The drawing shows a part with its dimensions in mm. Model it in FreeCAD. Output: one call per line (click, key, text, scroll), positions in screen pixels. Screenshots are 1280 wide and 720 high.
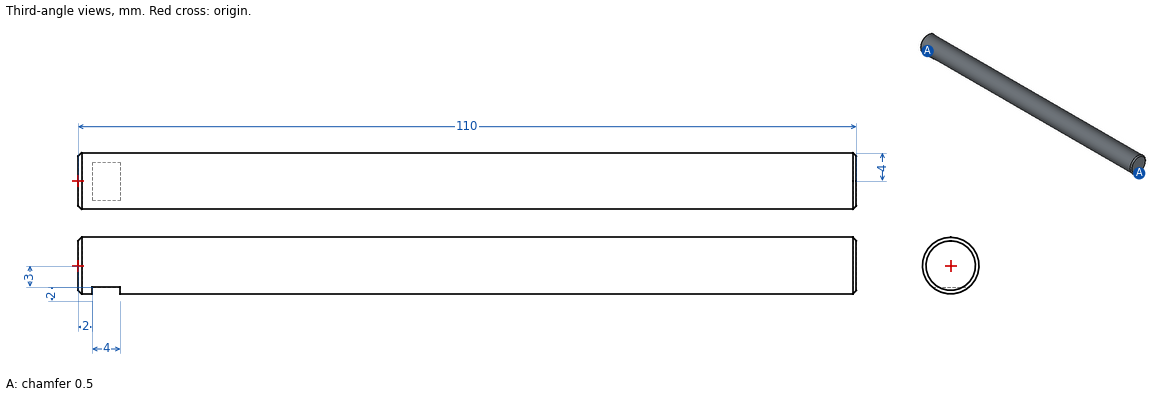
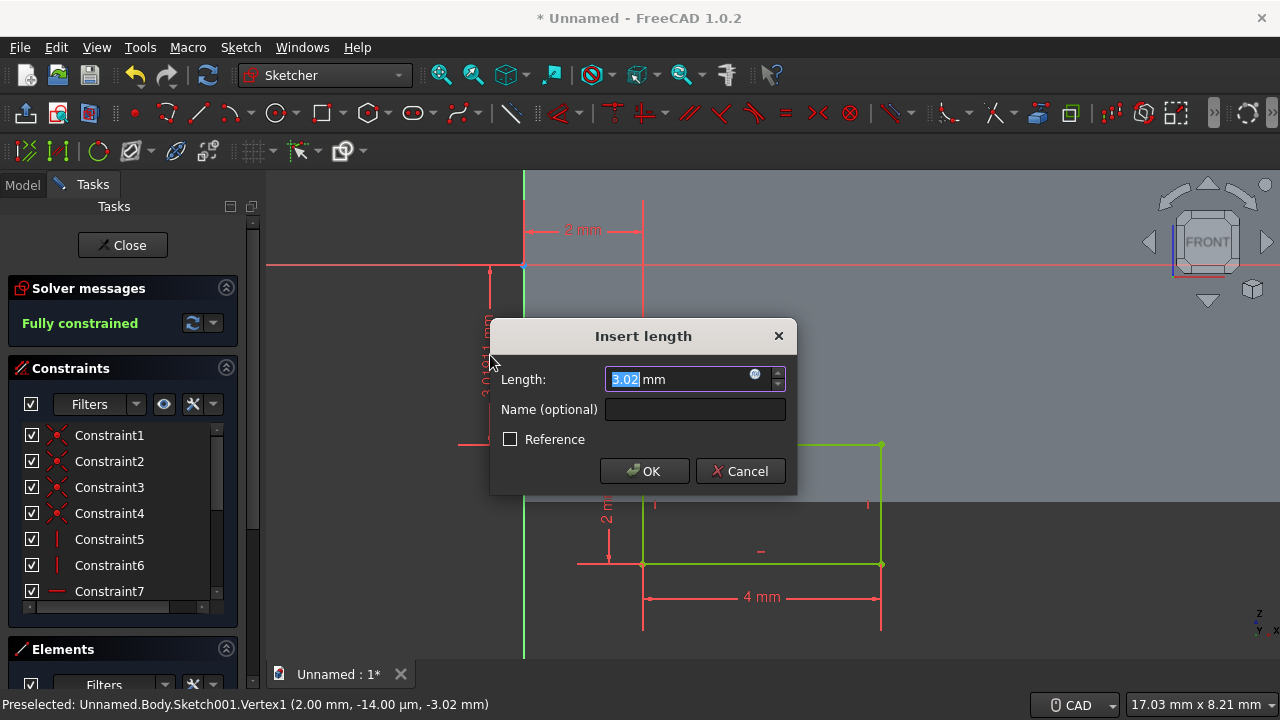
text(3)
key(Return)
key(Escape)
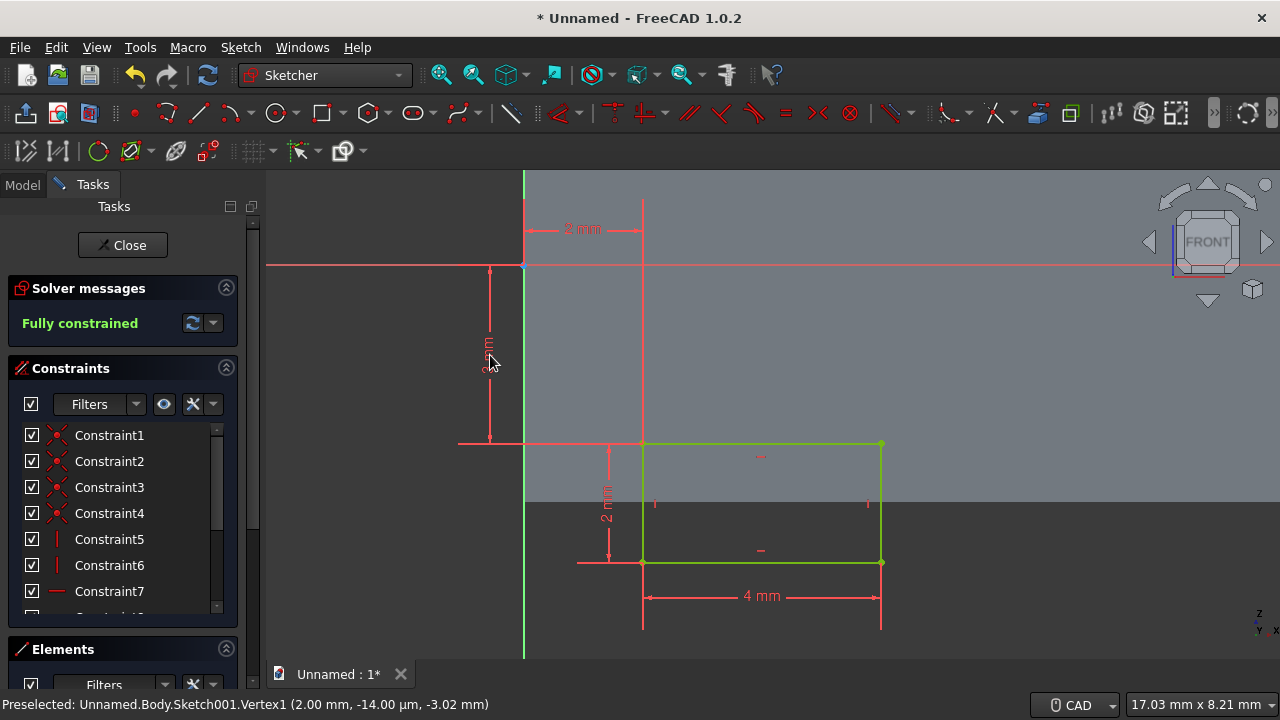
click(123, 245)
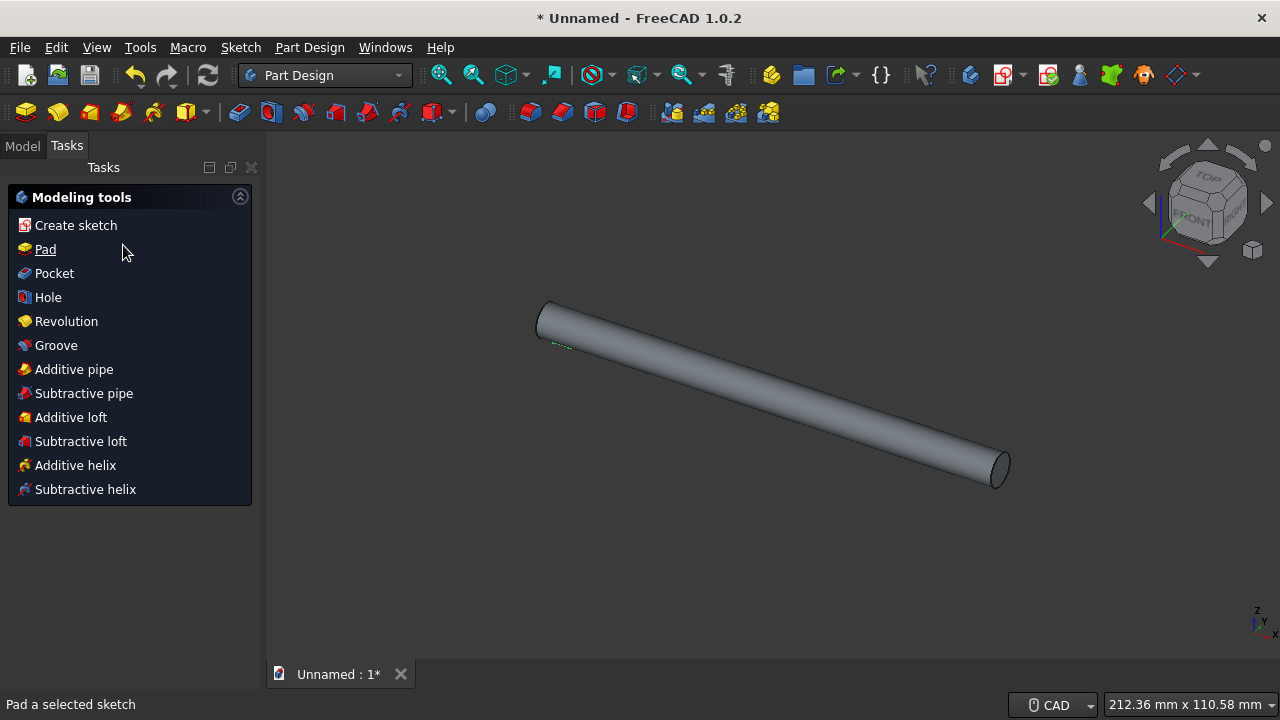
click(240, 112)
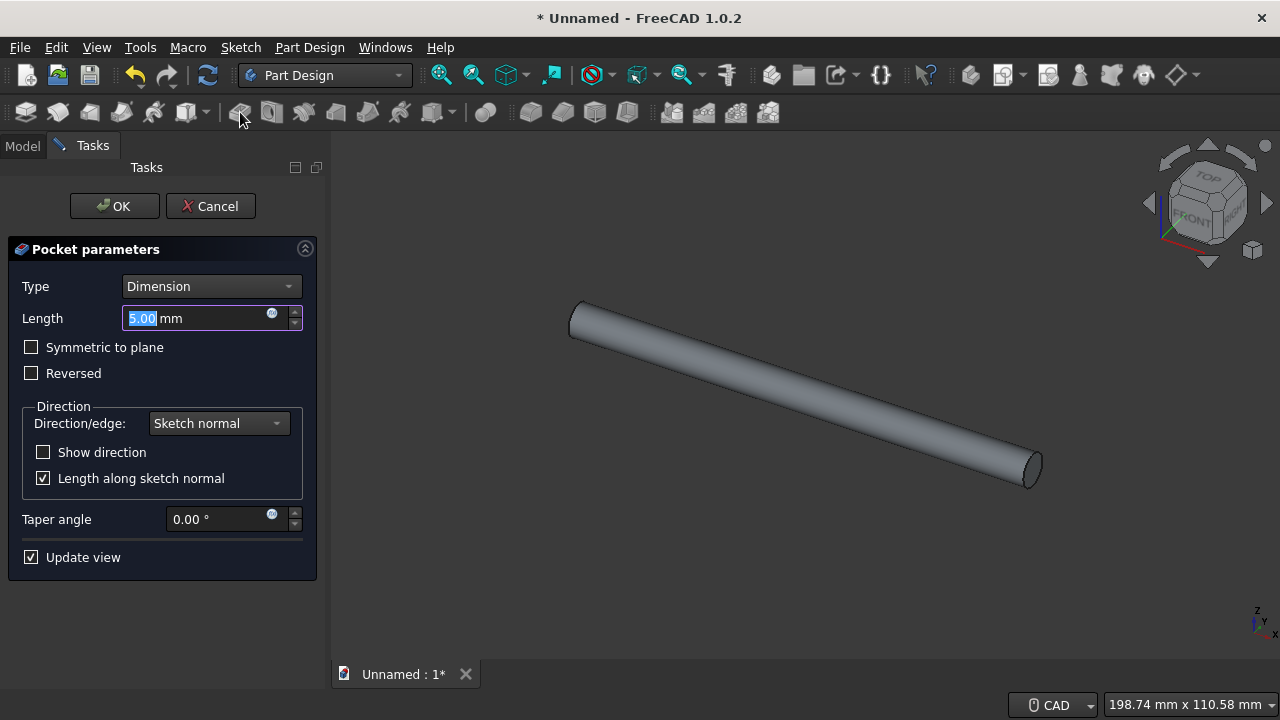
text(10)
key(Tab)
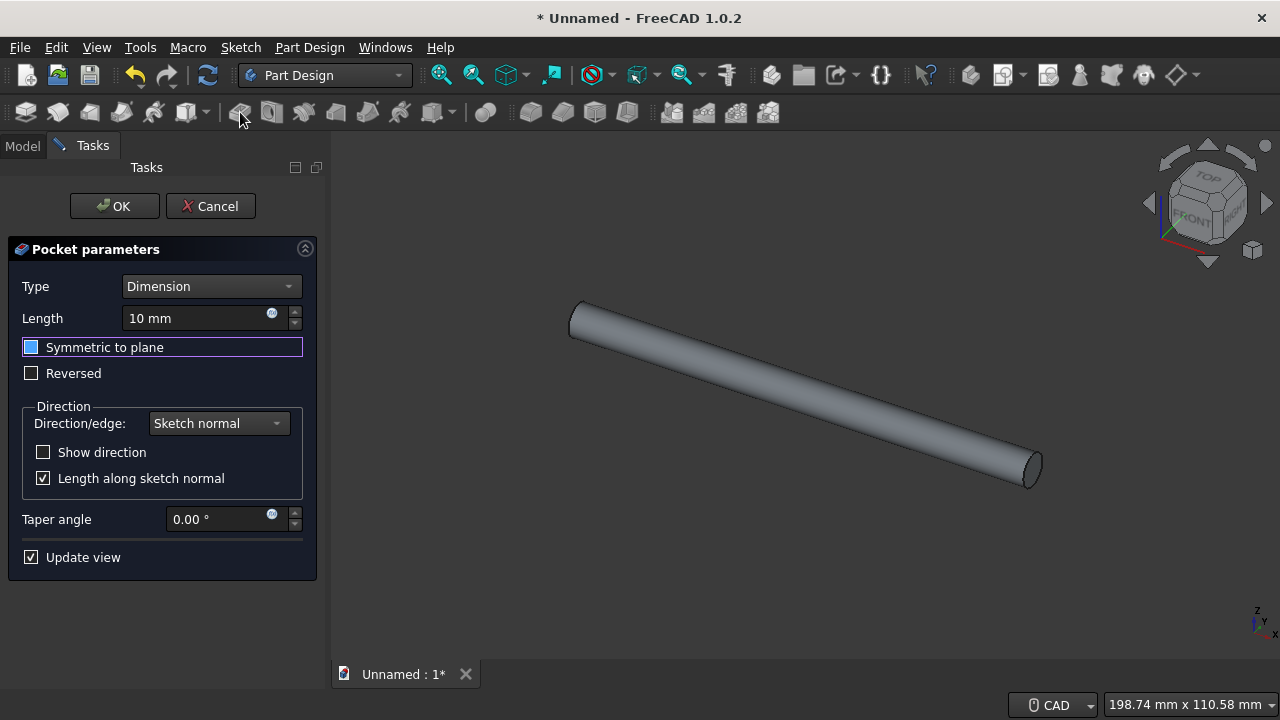
click(30, 347)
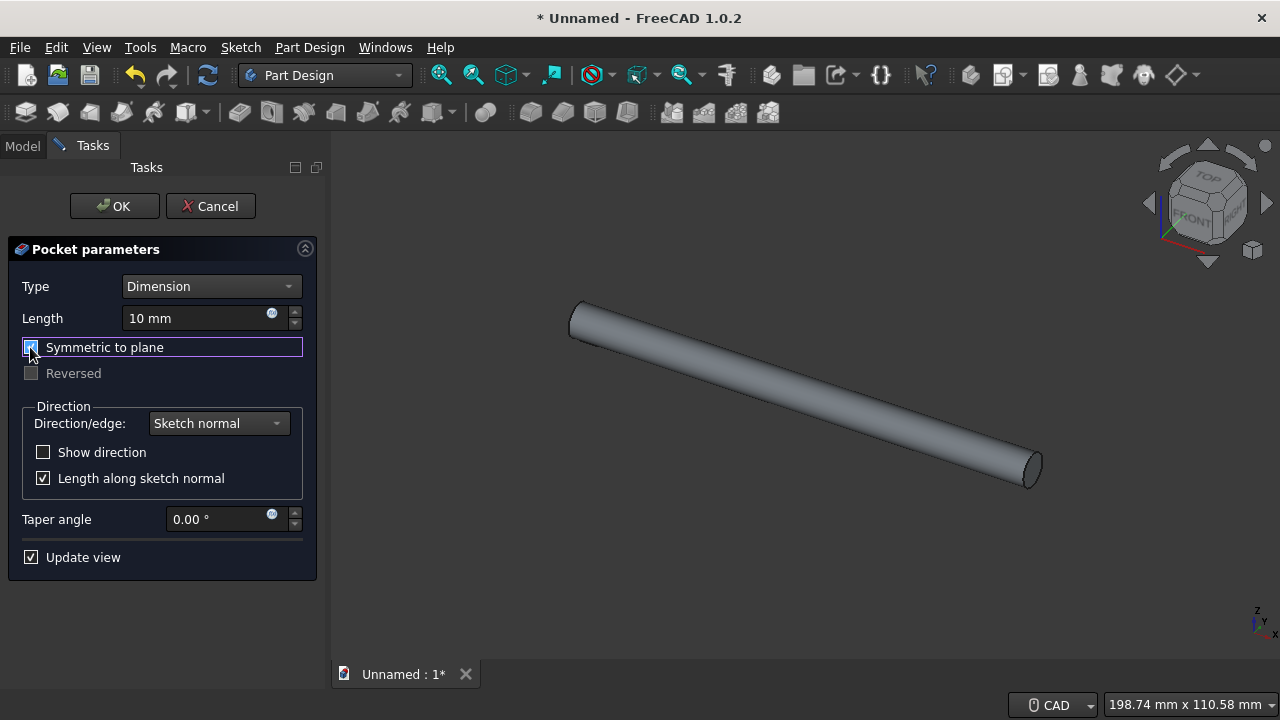
click(115, 206)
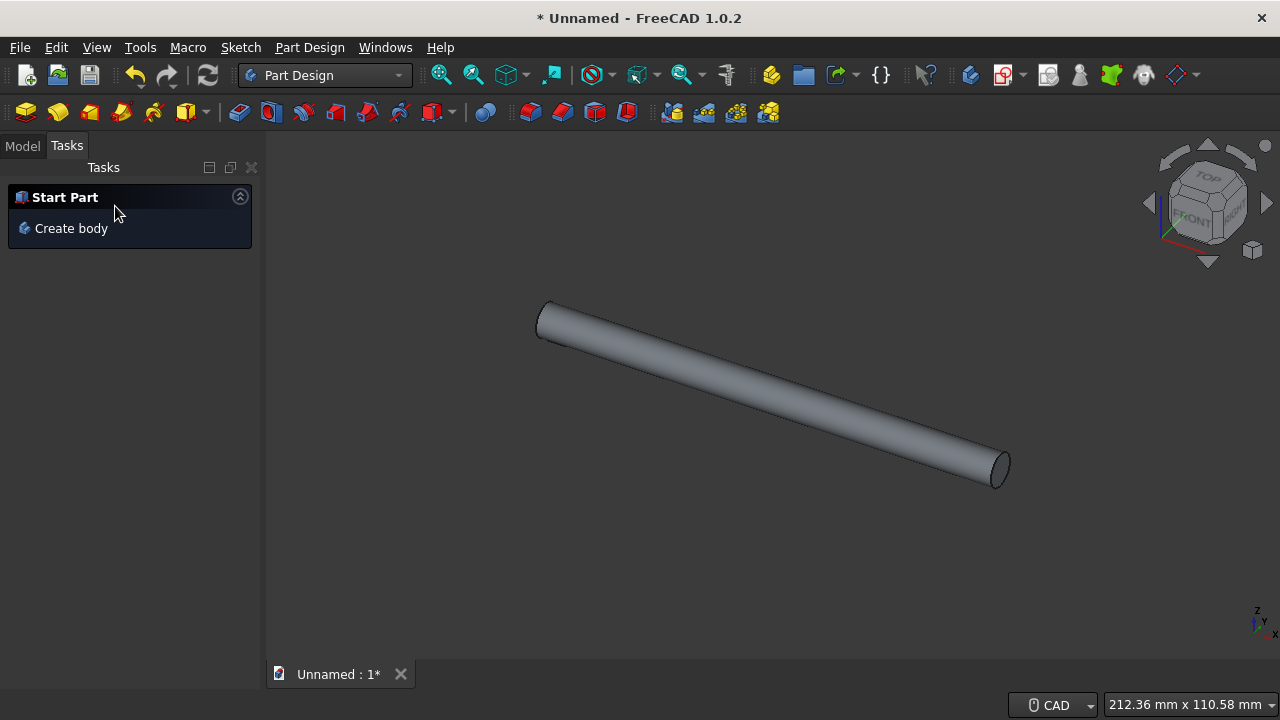
click(991, 479)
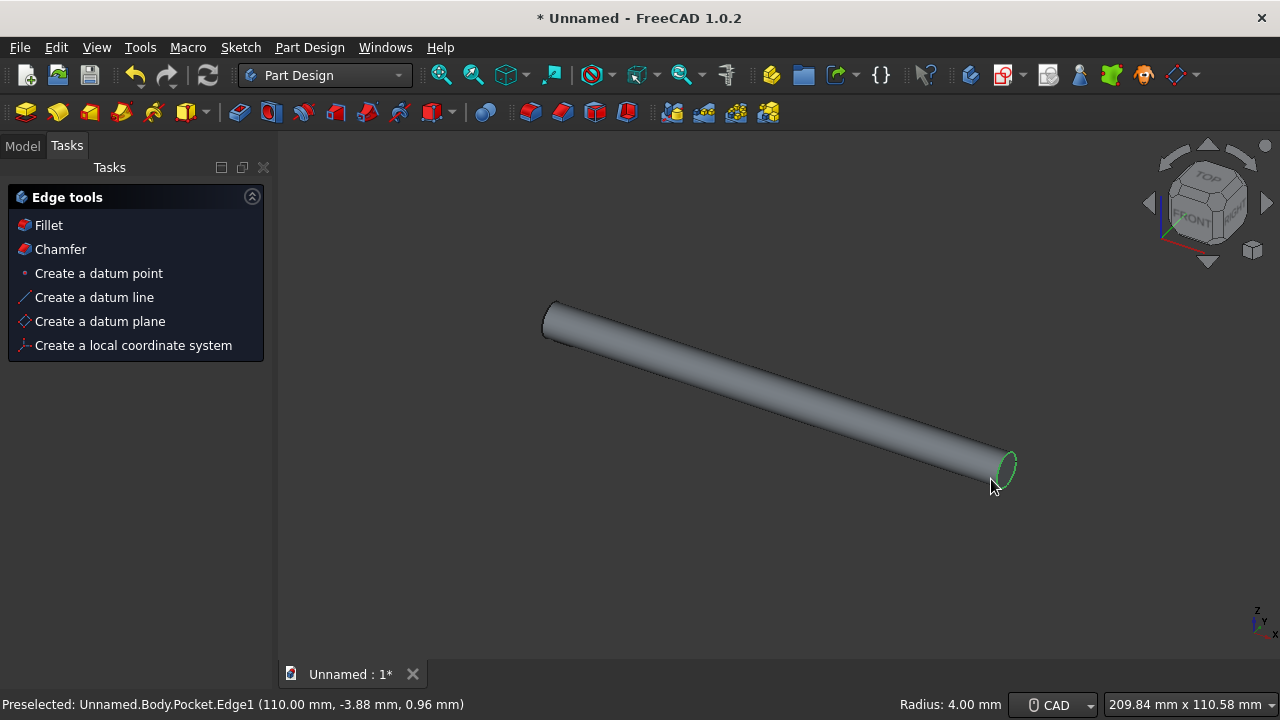
click(542, 328, ctrl)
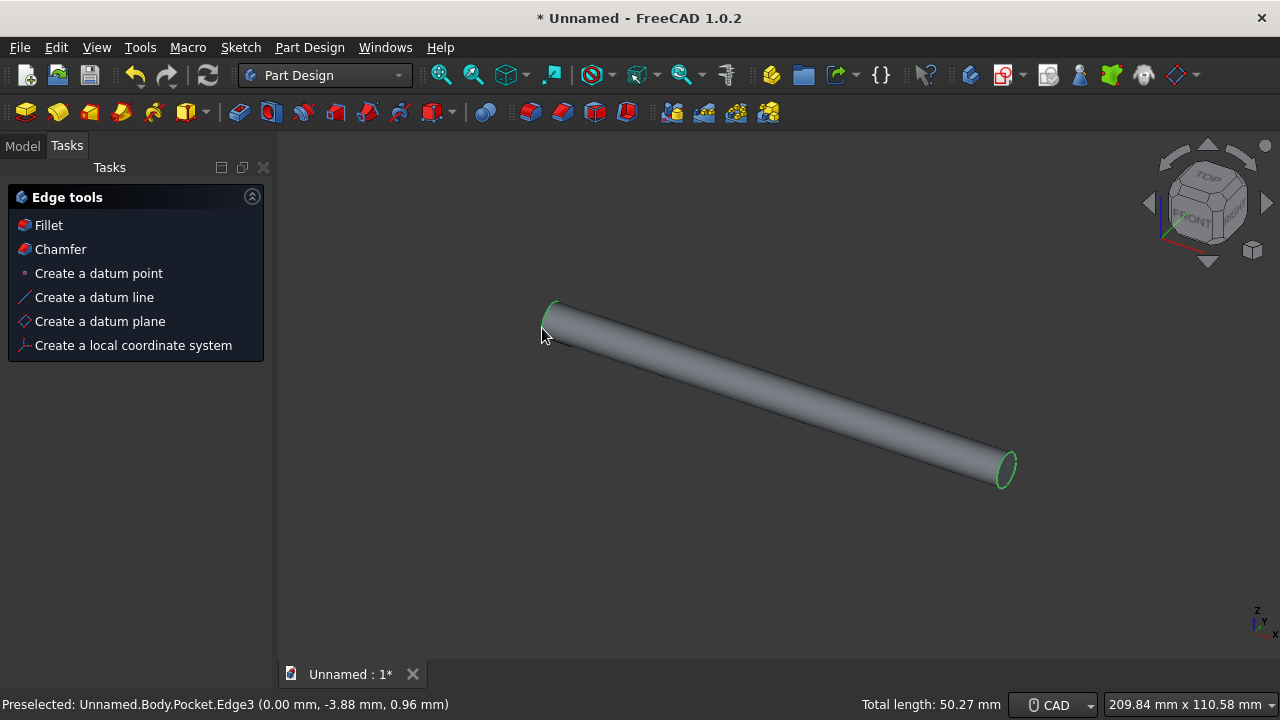
click(564, 112)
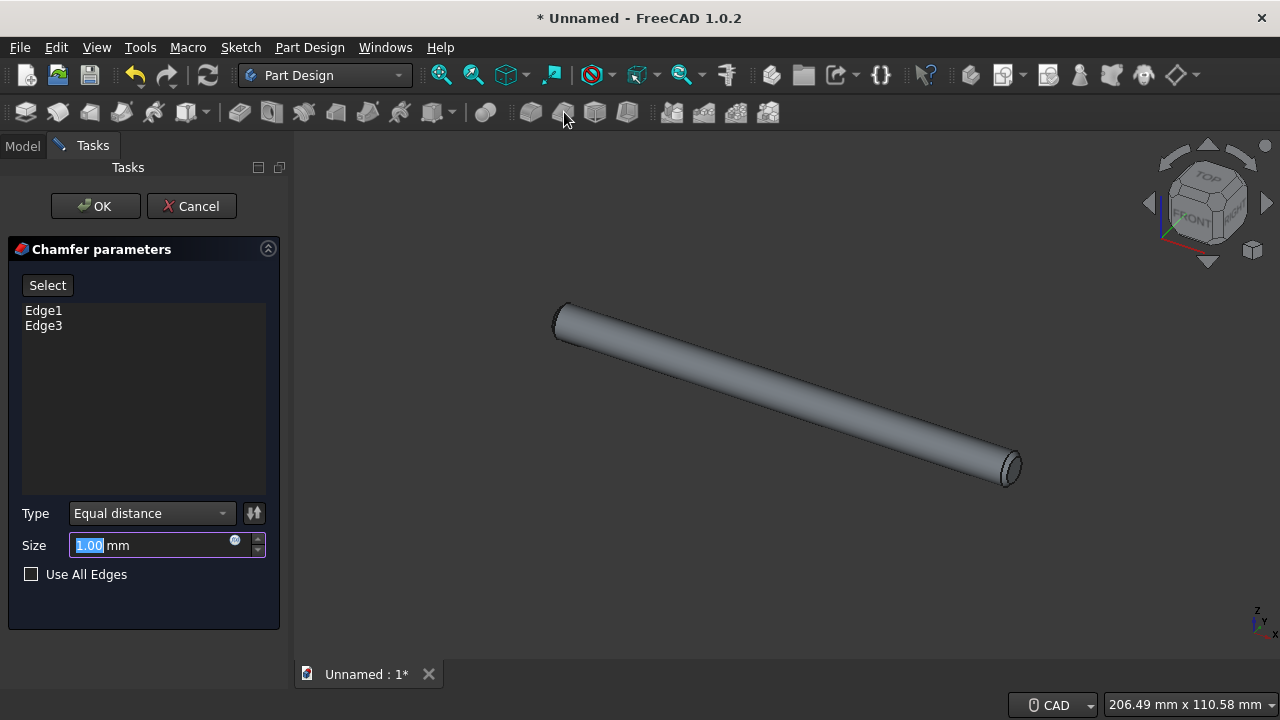
text(0.5)
key(Tab)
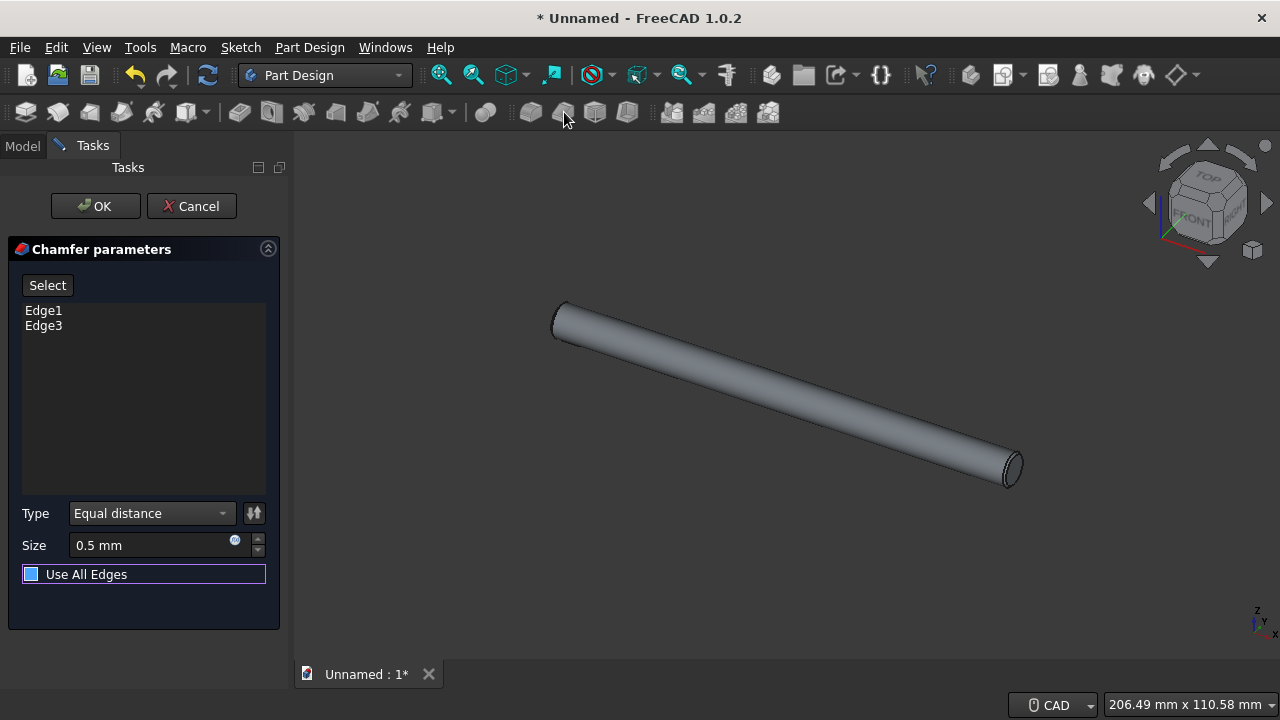
click(96, 206)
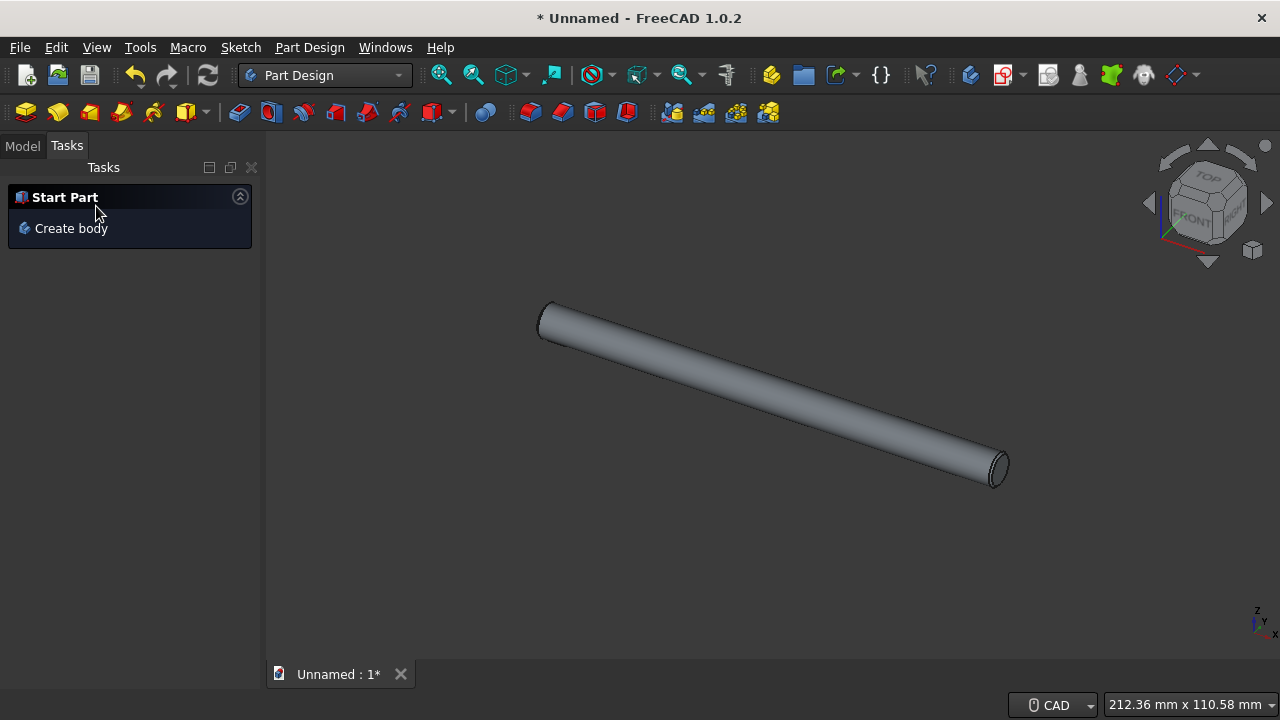
key(0)